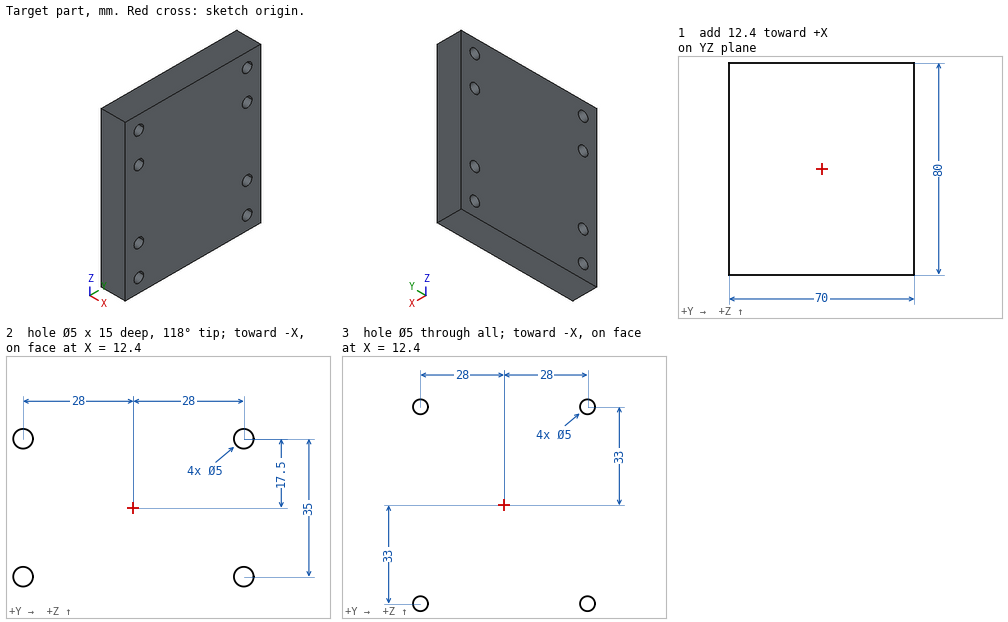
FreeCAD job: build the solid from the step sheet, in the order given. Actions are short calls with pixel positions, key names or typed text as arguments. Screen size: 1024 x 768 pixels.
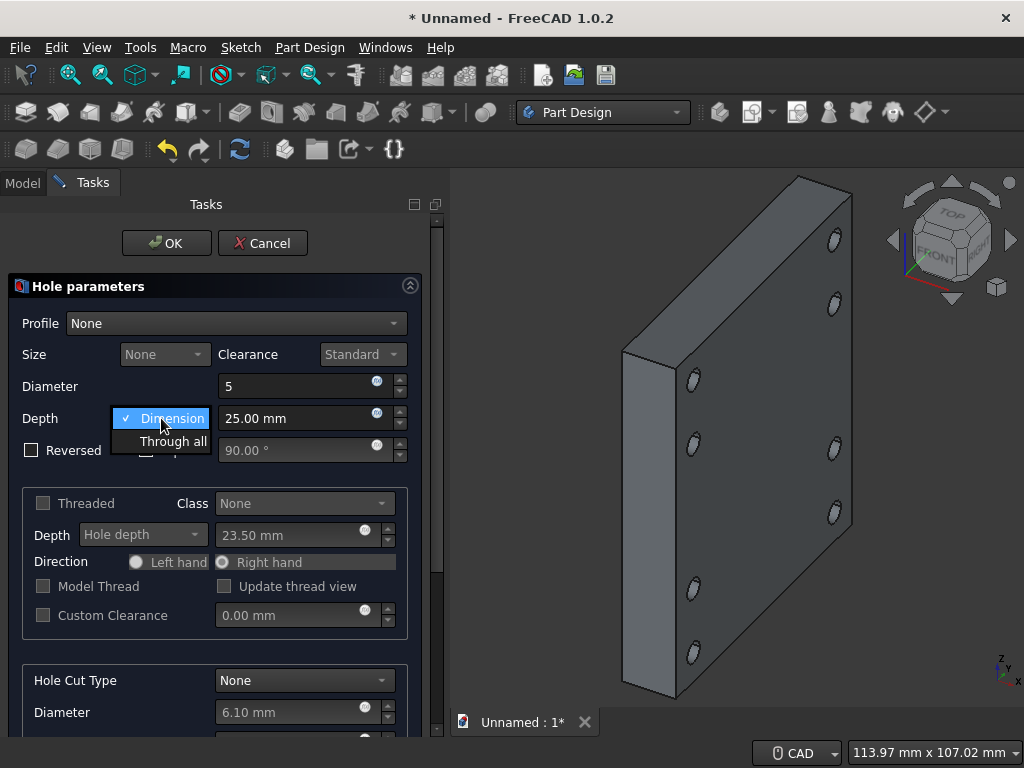
click(160, 442)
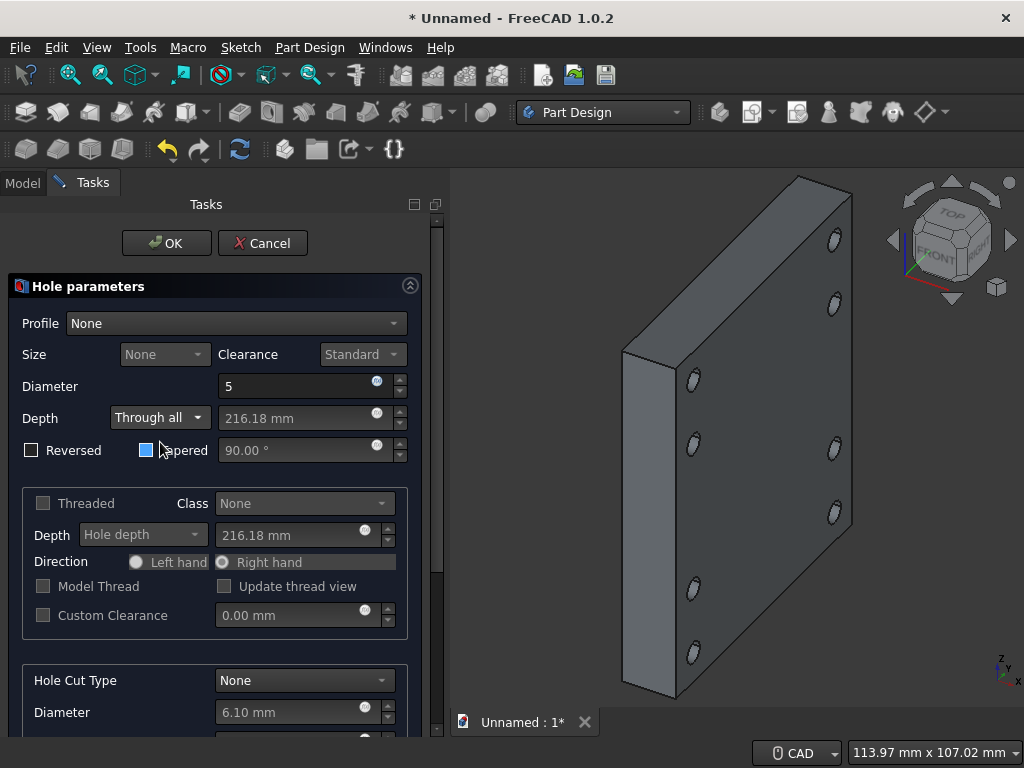
click(167, 243)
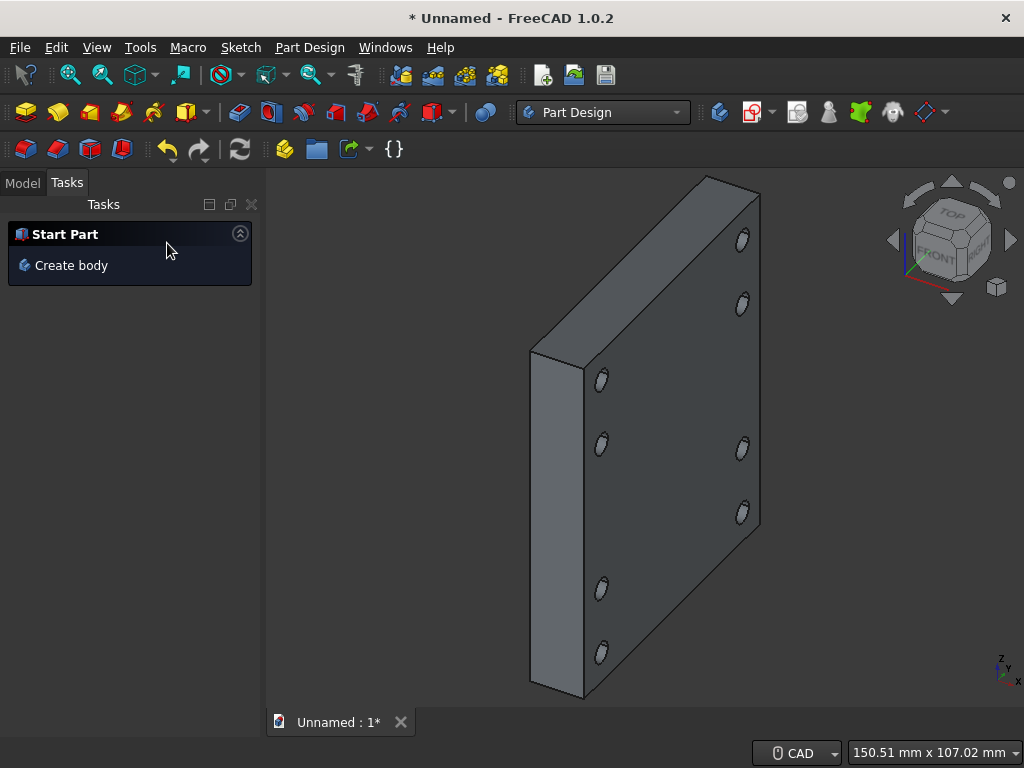
key(0)